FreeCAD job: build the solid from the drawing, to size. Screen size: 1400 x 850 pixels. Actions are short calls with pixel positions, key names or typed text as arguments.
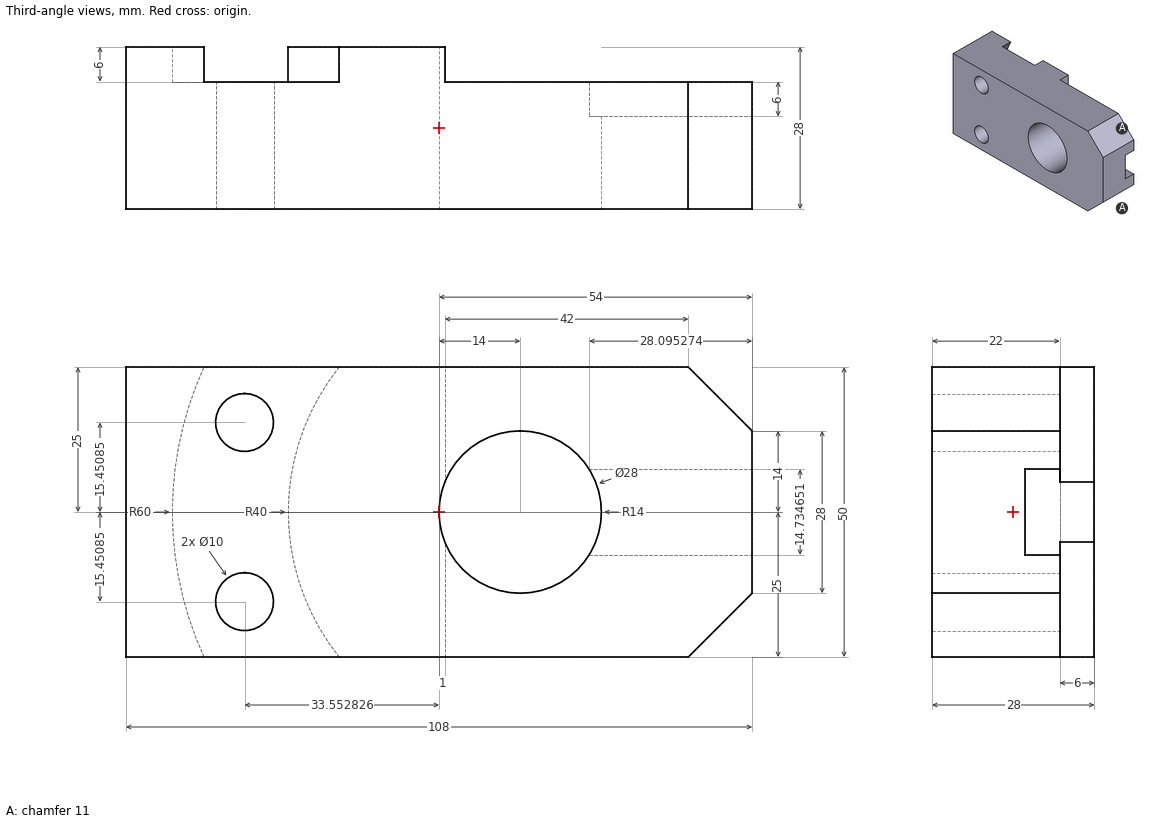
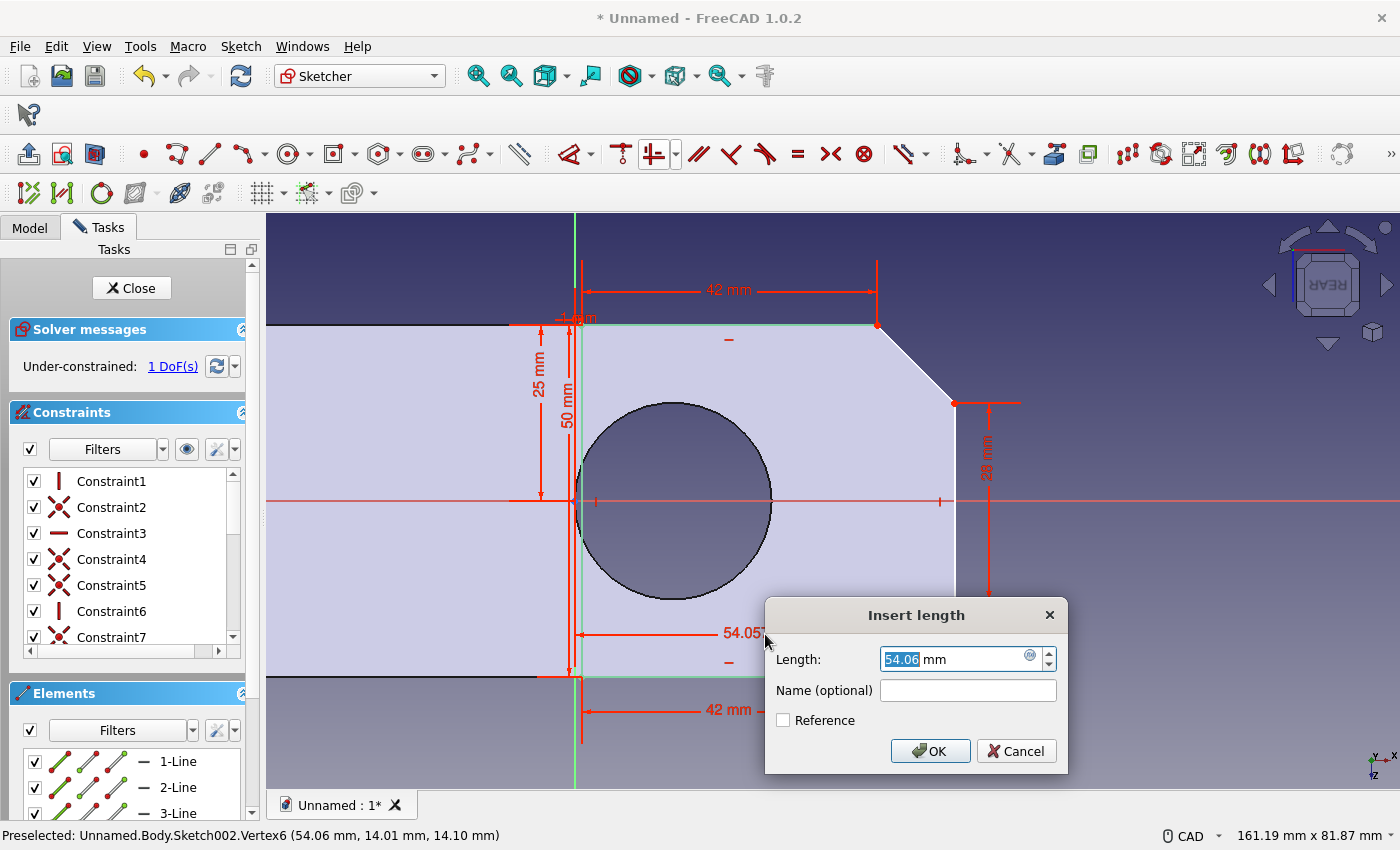
text(54)
key(Return)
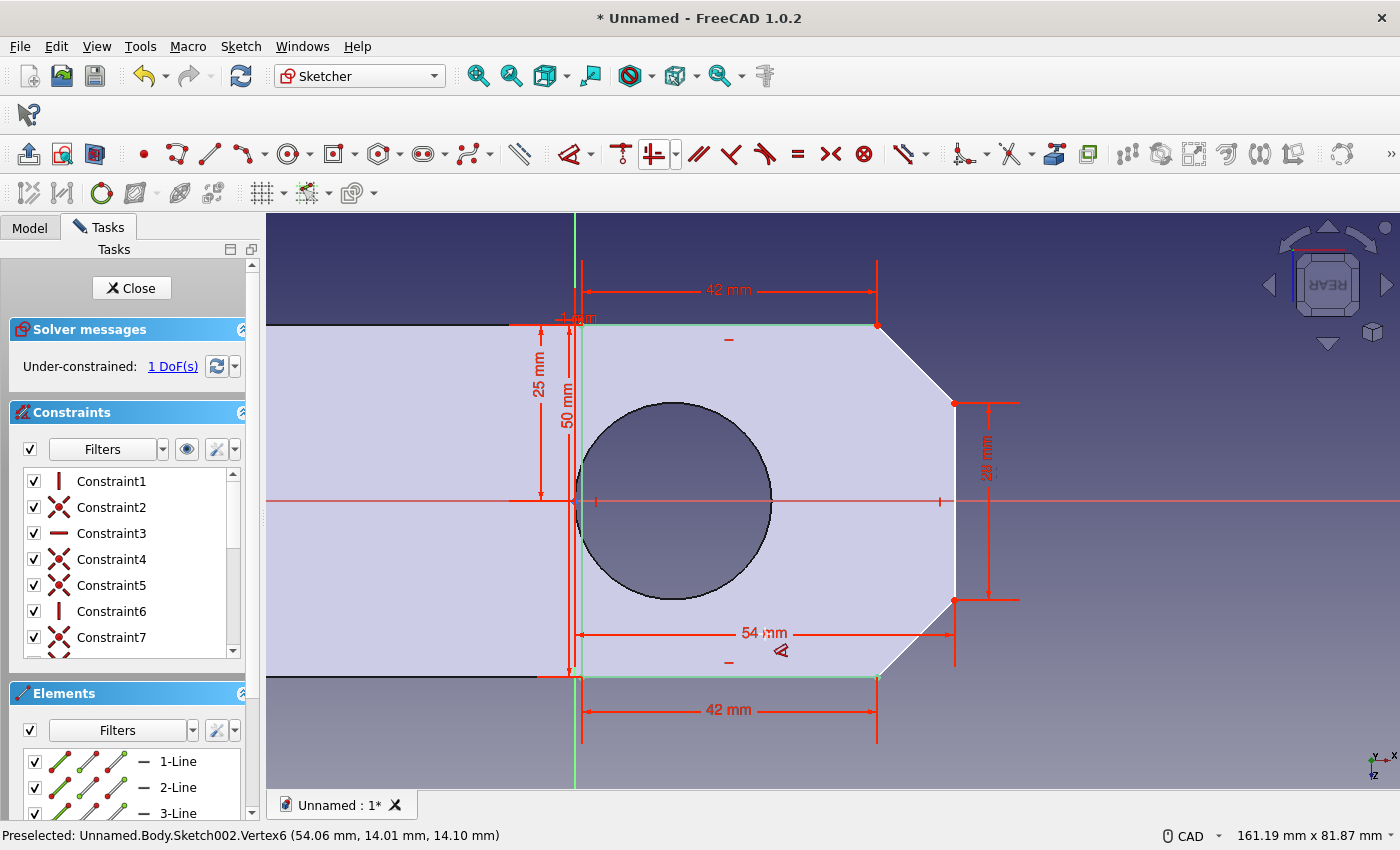
click(955, 600)
click(989, 551)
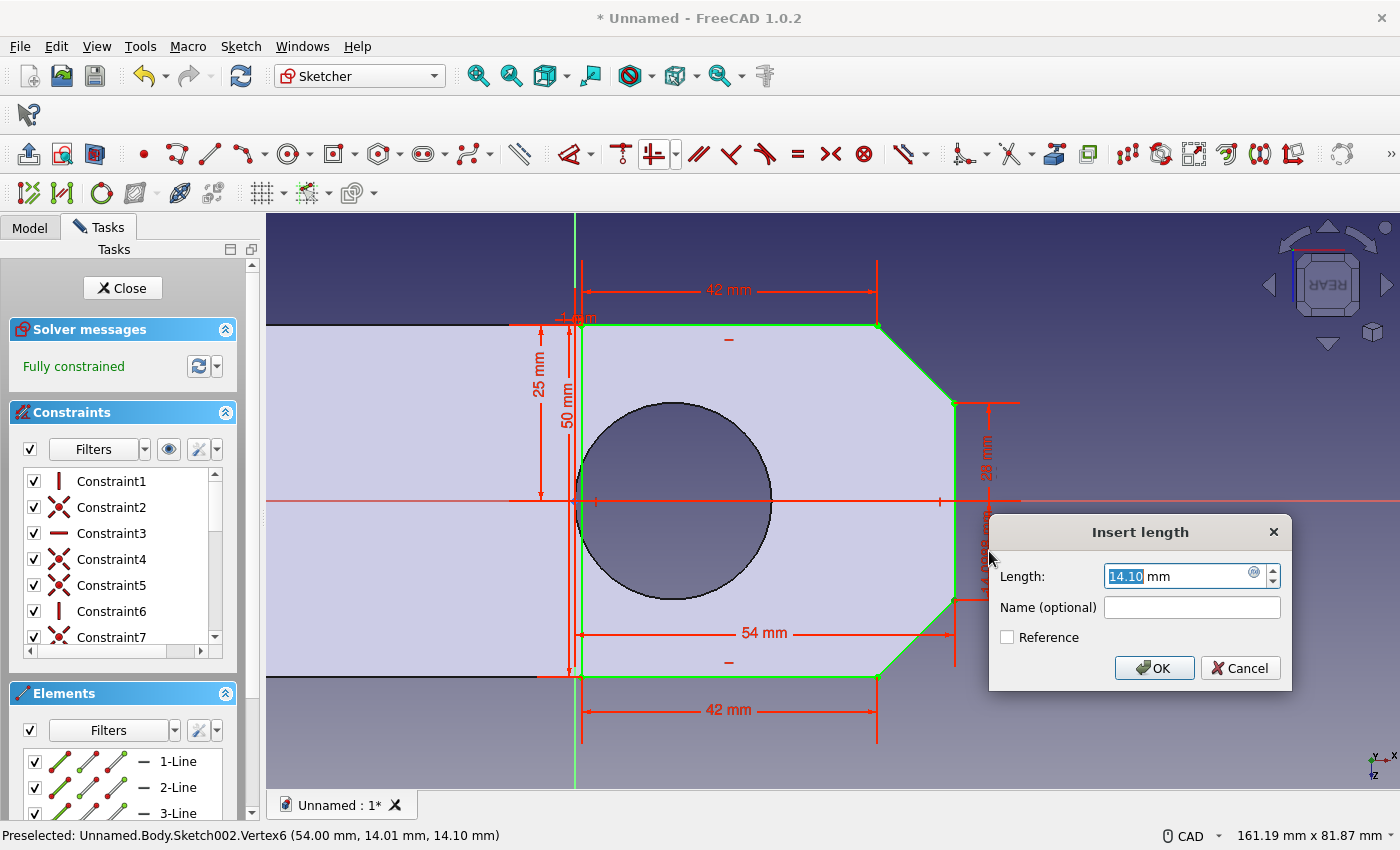
text(14)
key(Return)
key(Escape)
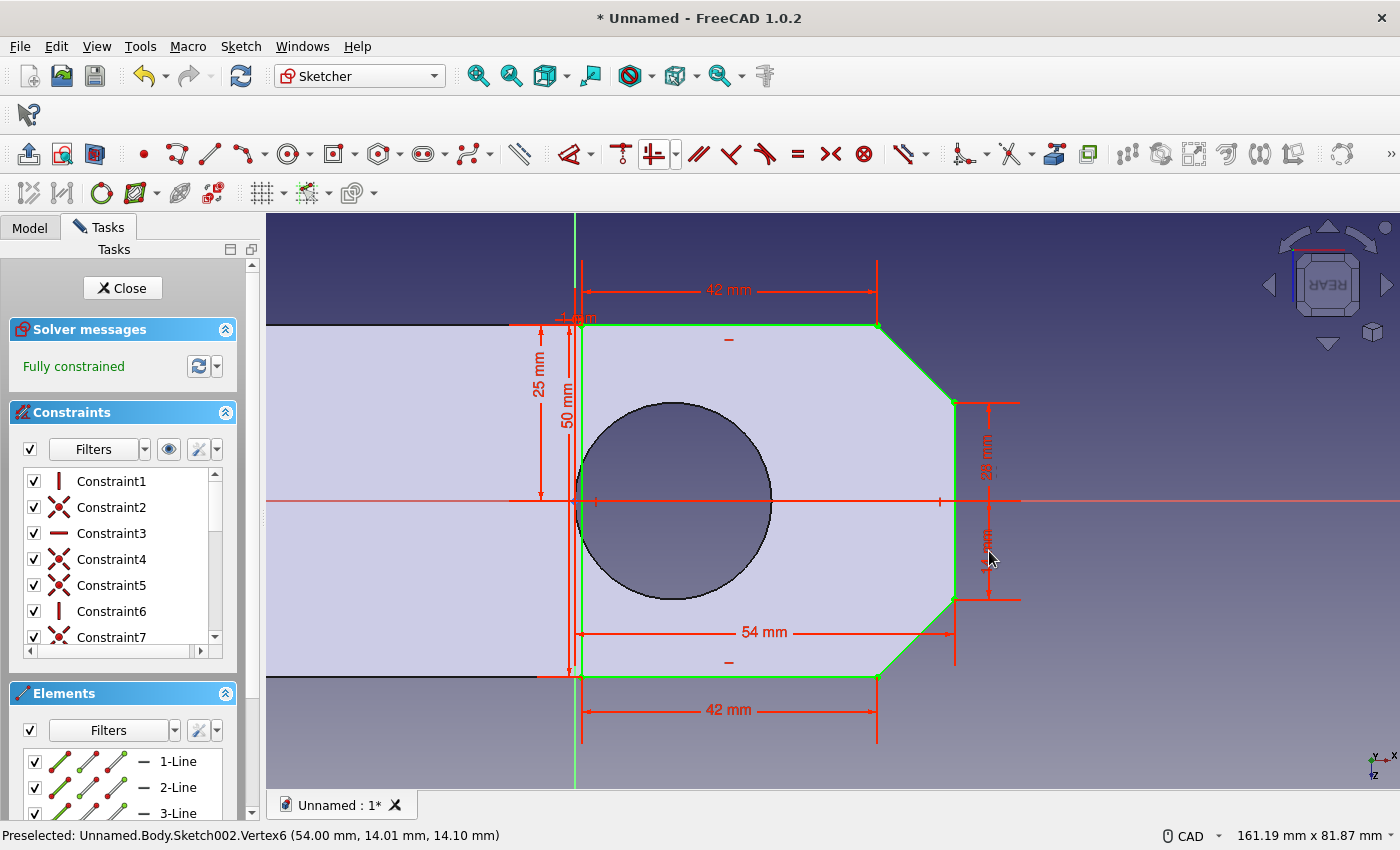
click(123, 288)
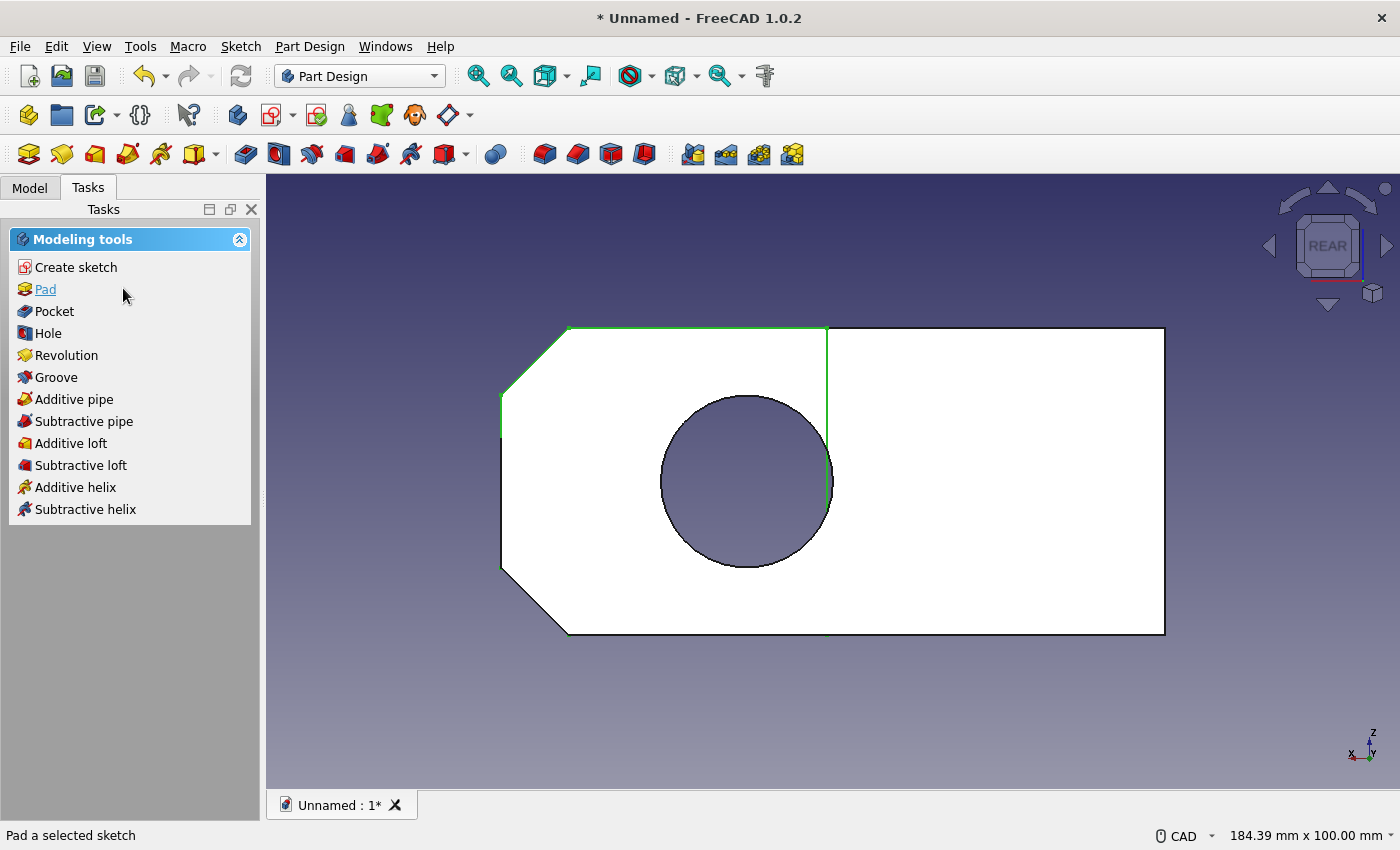
click(246, 154)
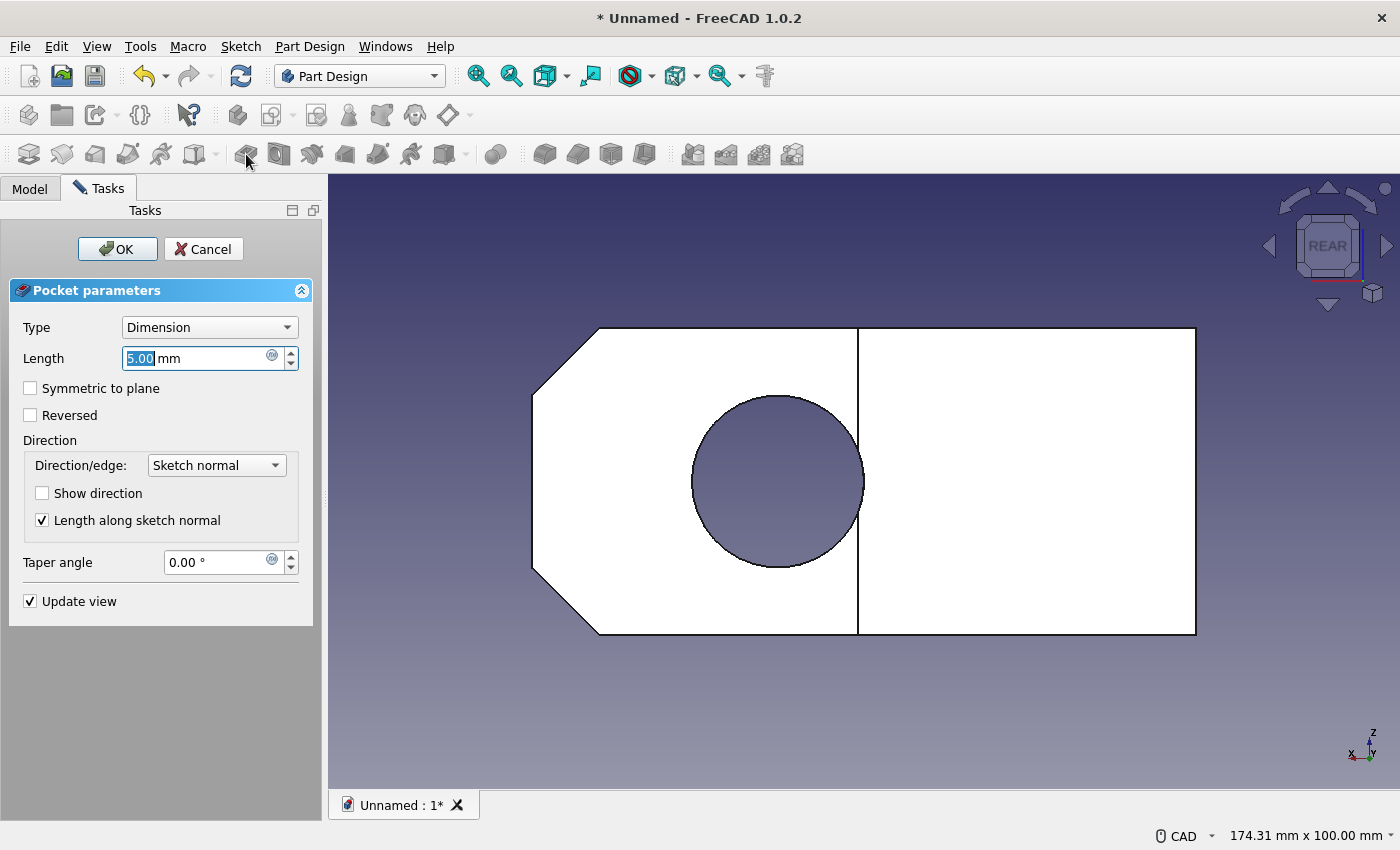
text(6)
key(Tab)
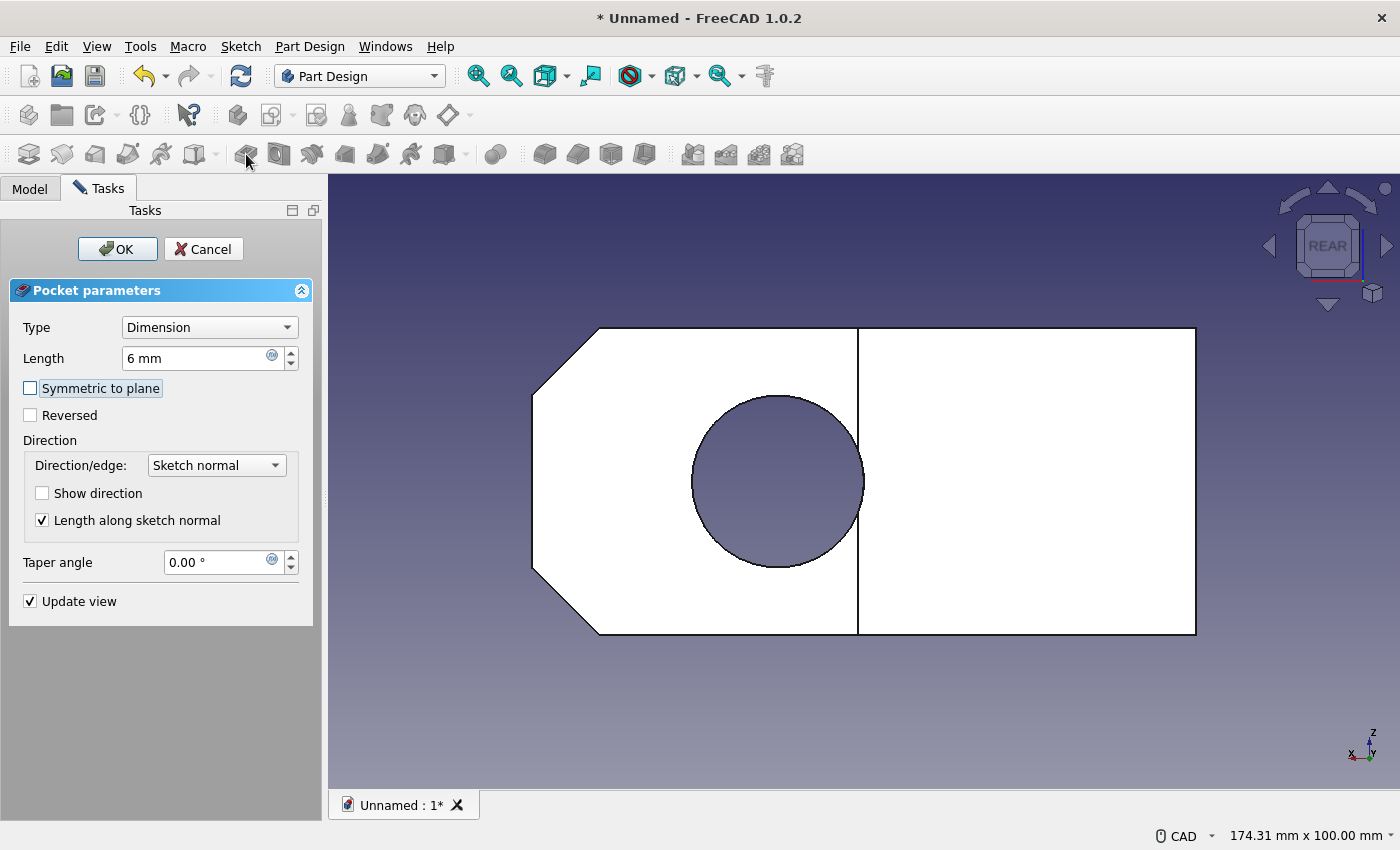
click(118, 249)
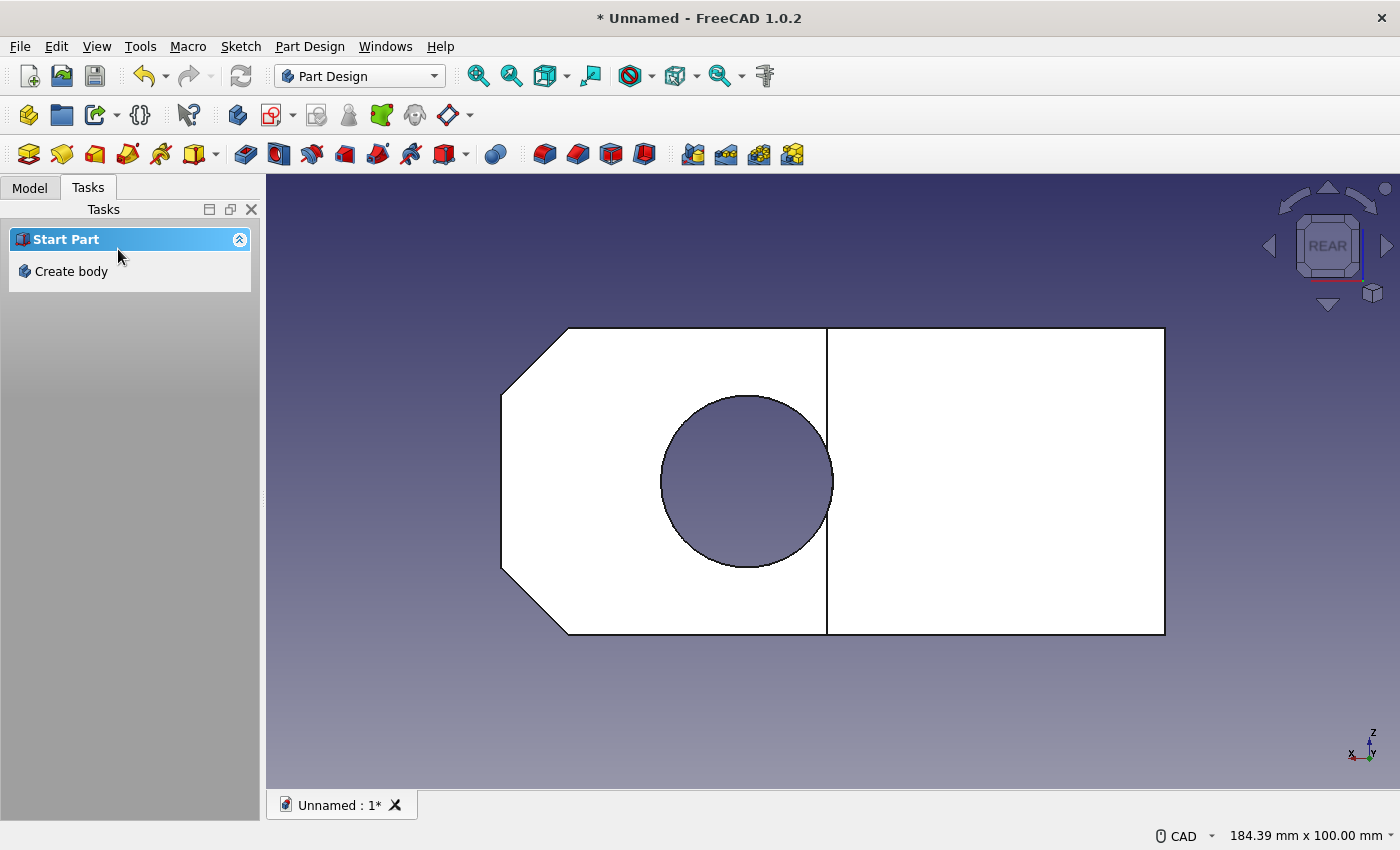
click(996, 480)